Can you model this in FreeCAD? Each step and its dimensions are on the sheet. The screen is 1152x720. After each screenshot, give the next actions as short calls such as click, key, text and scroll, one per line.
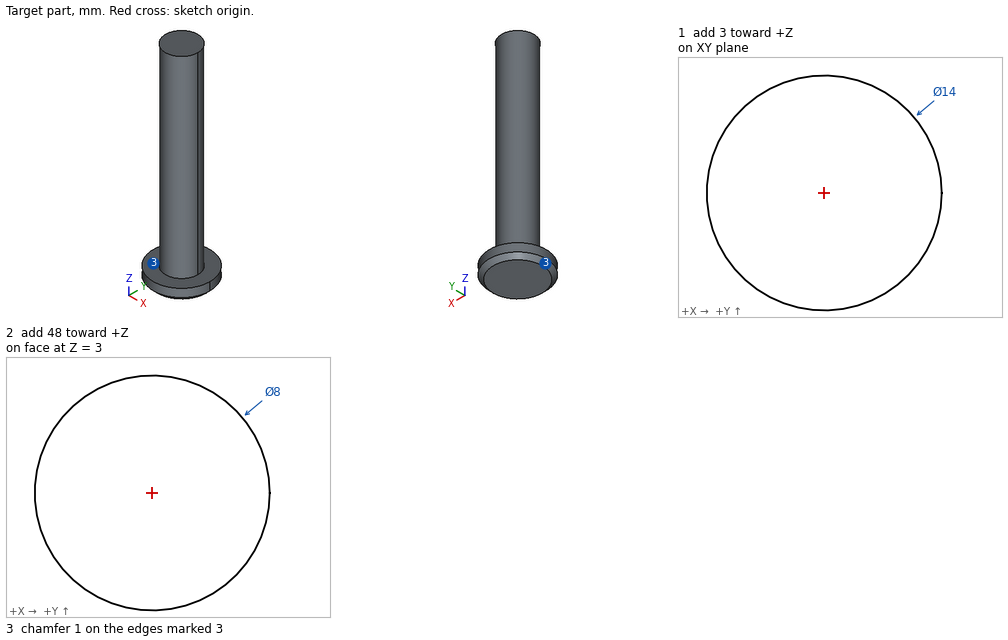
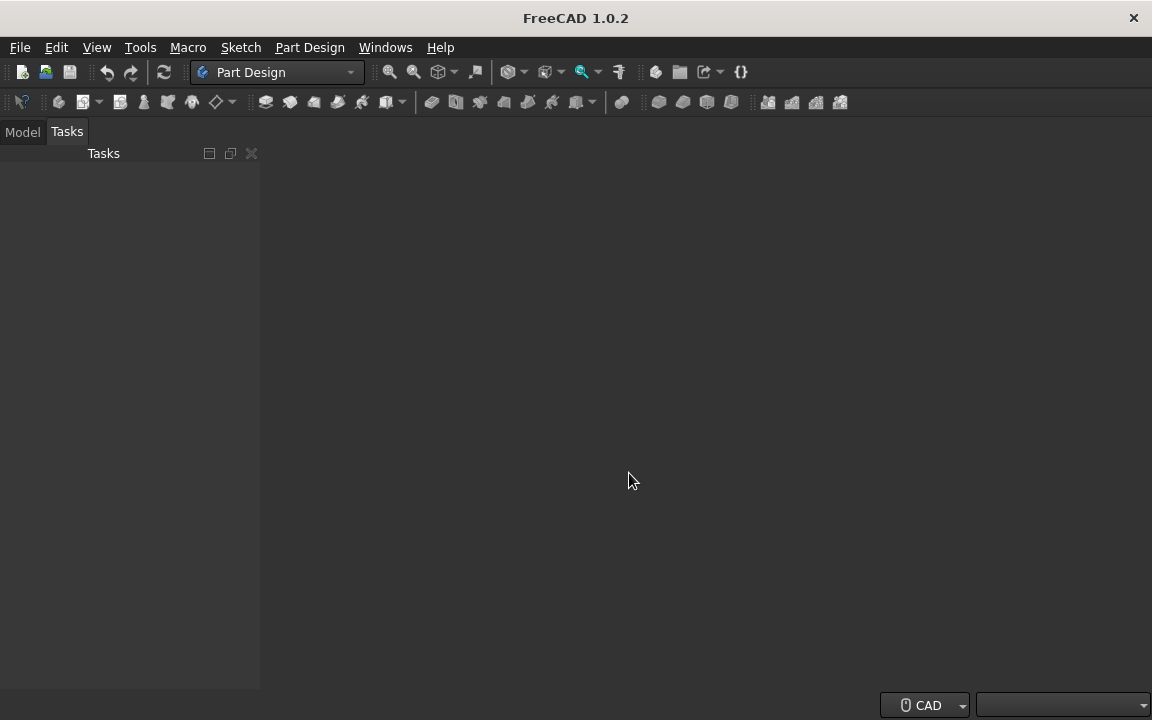
click(22, 72)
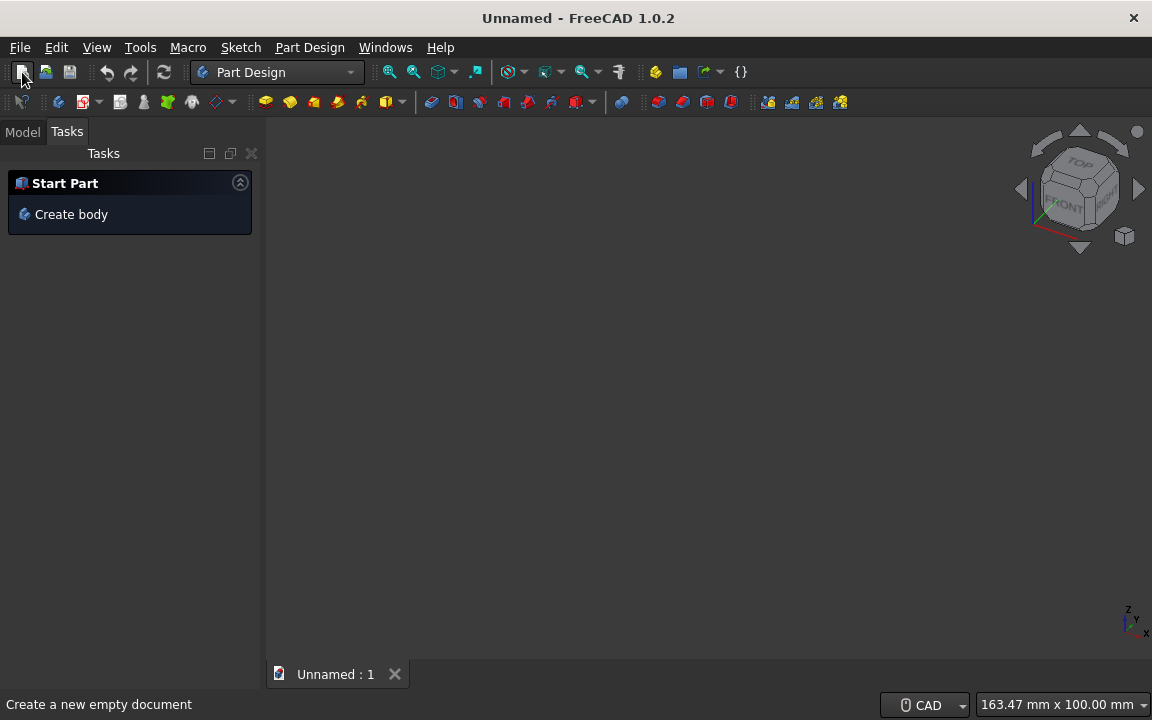
click(84, 102)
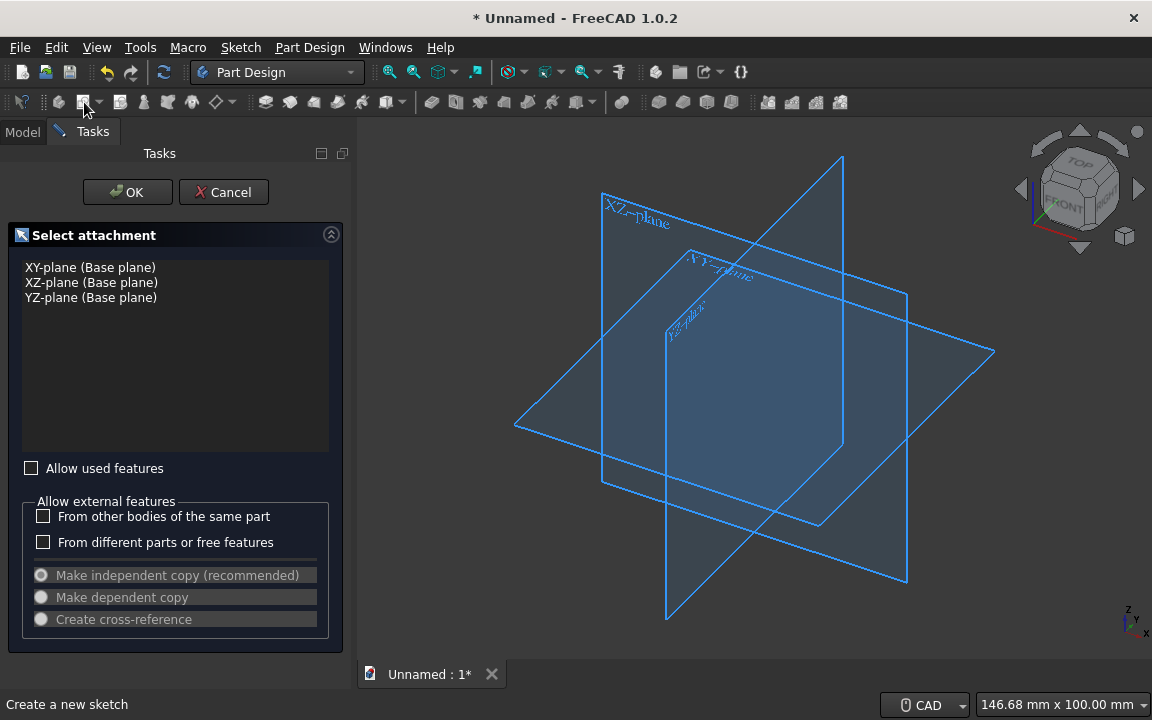
click(82, 268)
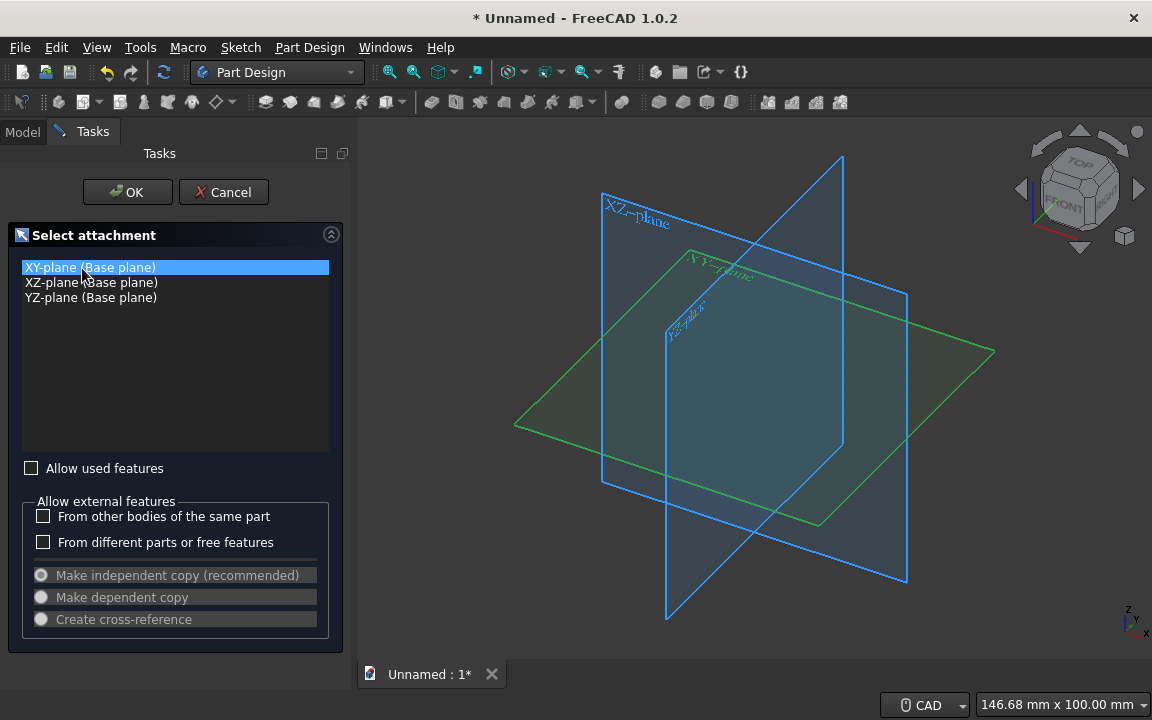
click(128, 192)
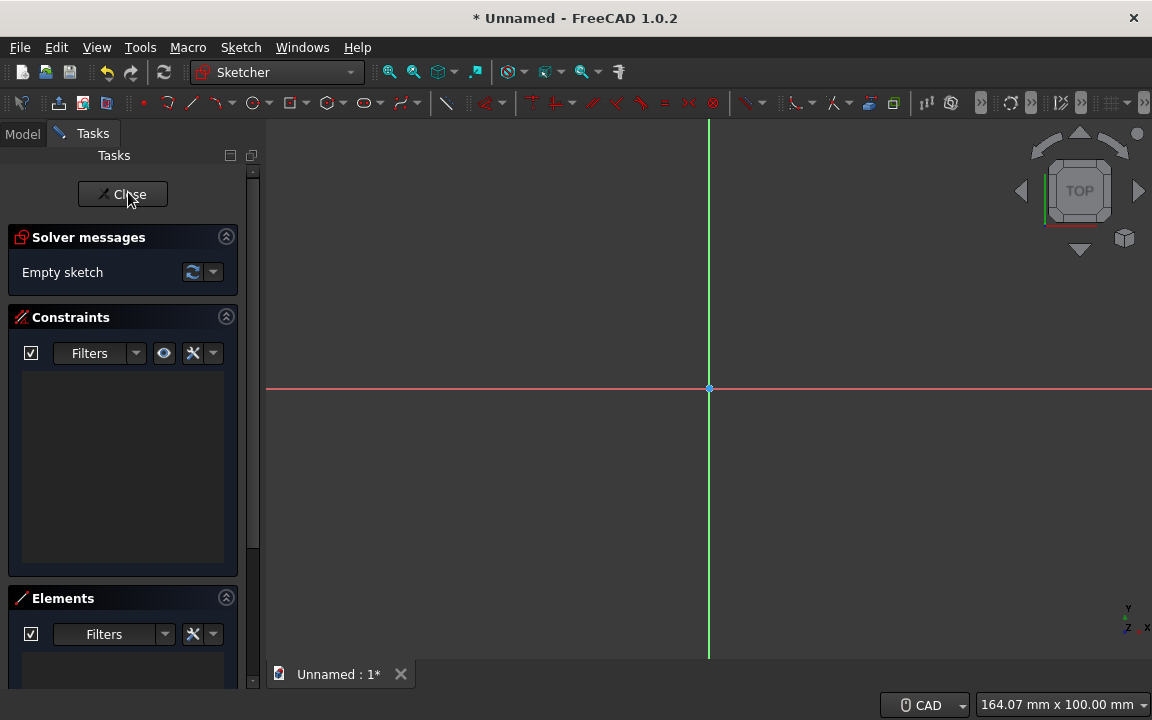
scroll(726, 389, up, 8)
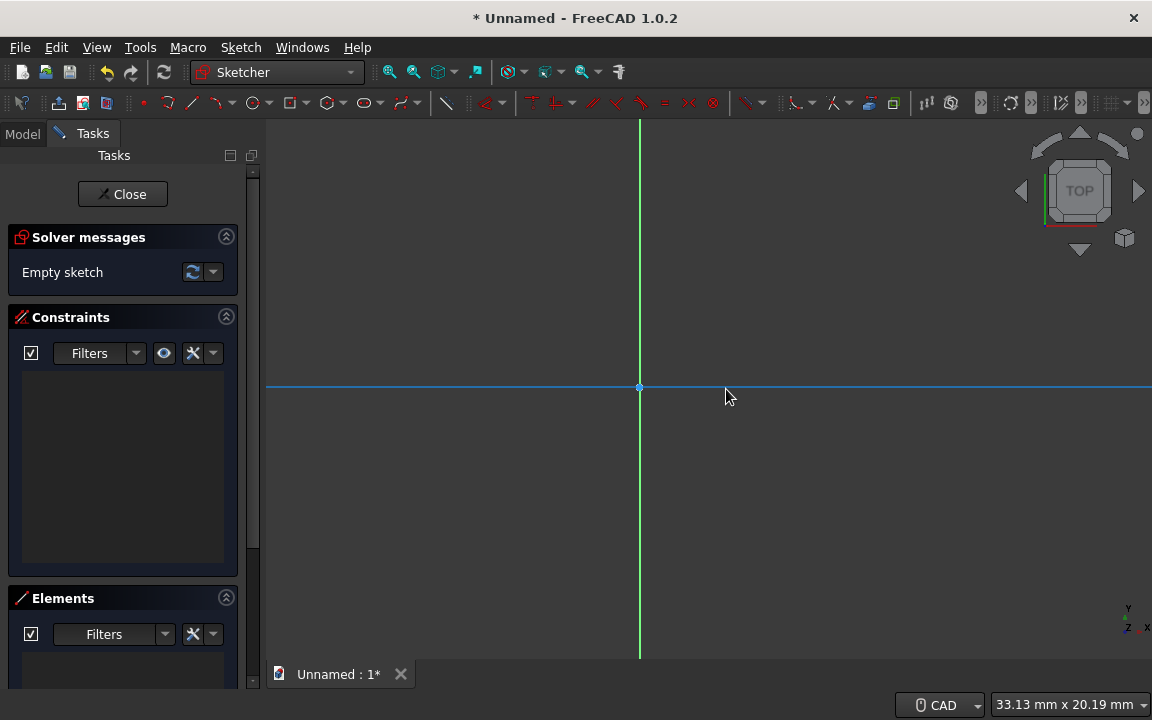
click(254, 104)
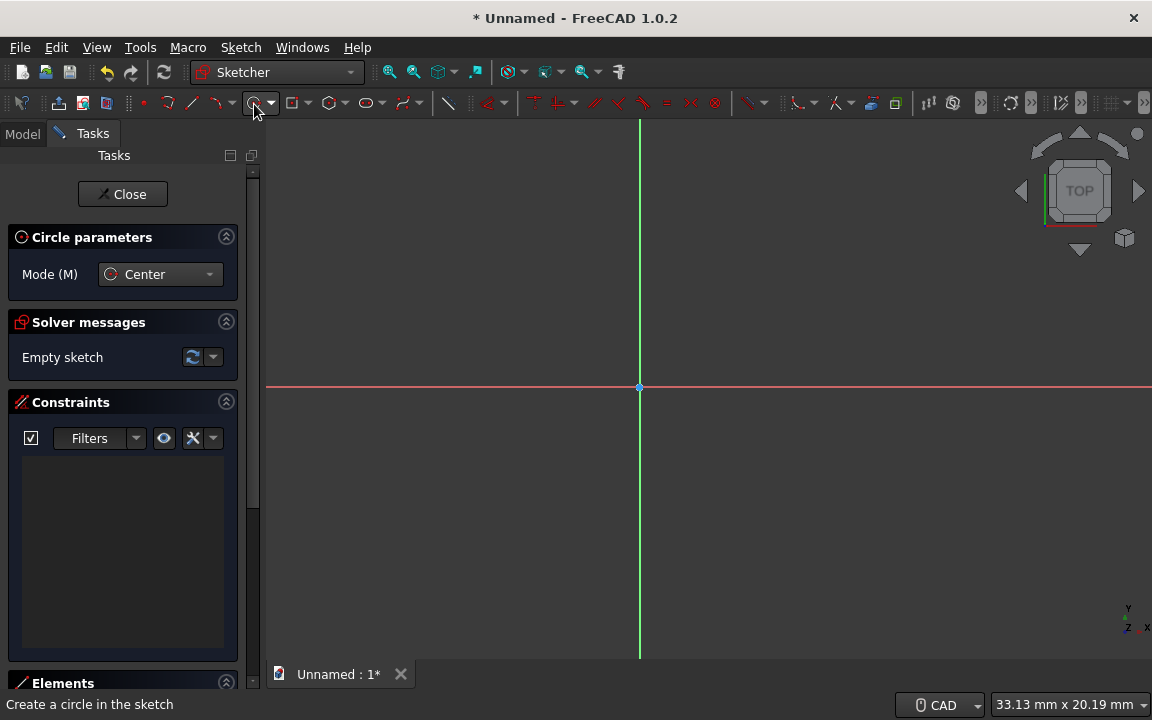
click(640, 387)
click(772, 255)
key(Escape)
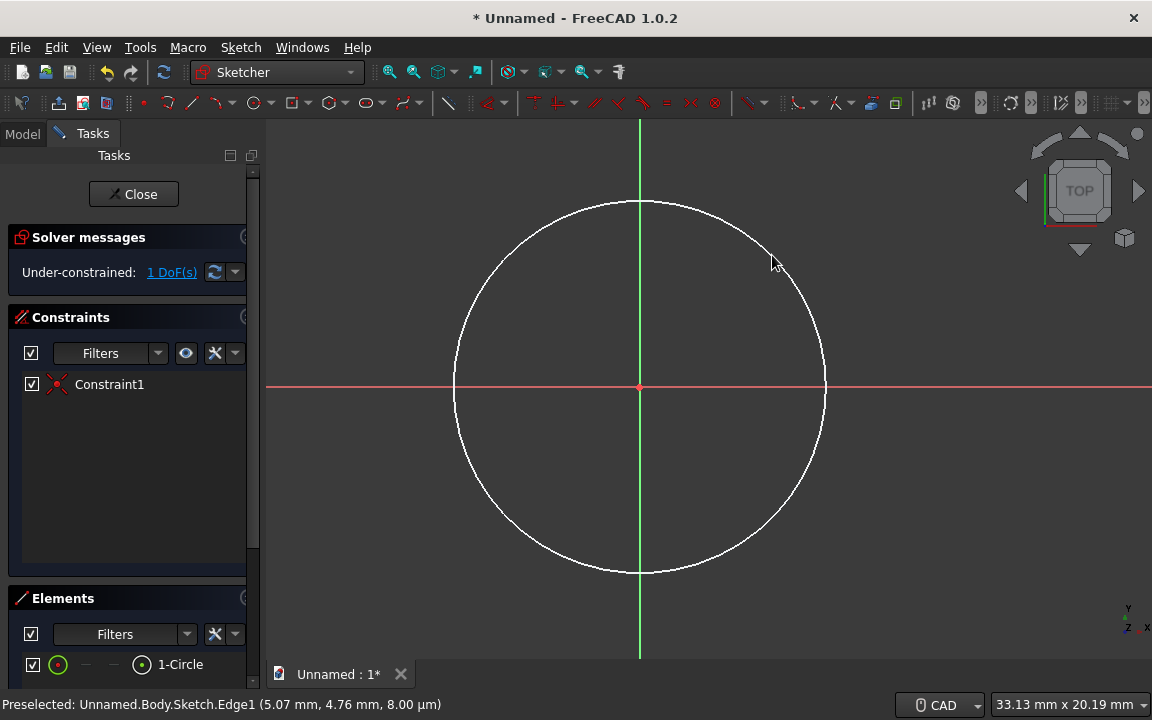
click(771, 255)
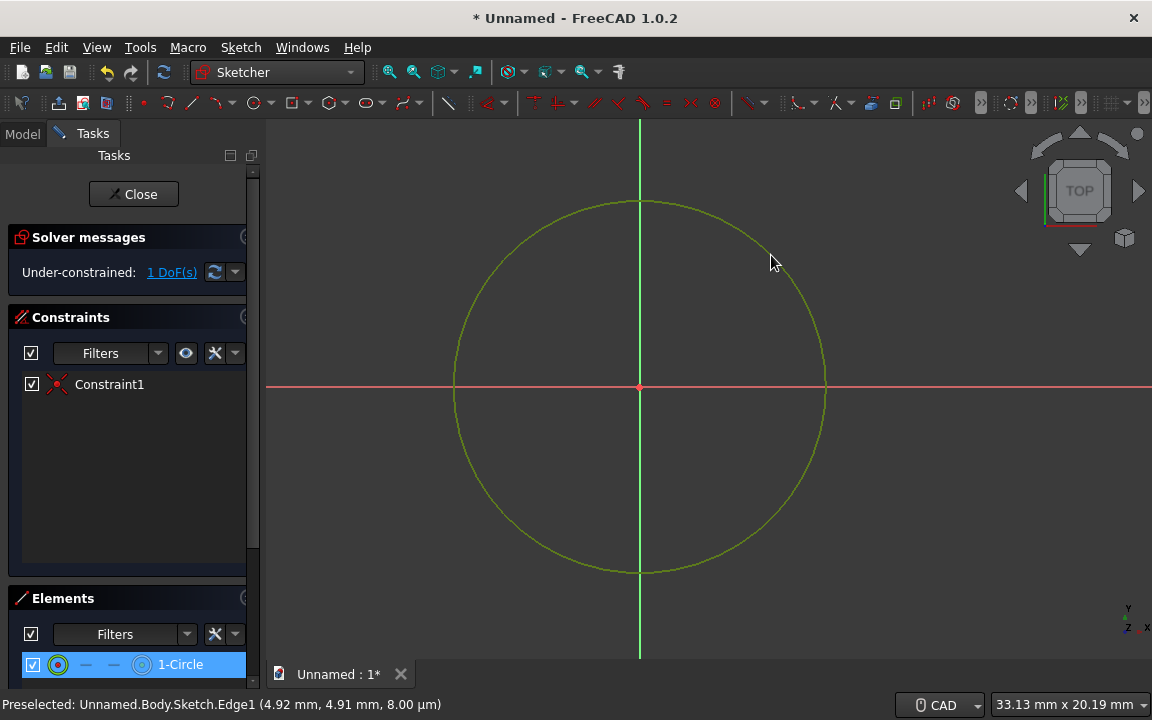
key(k)
key(o)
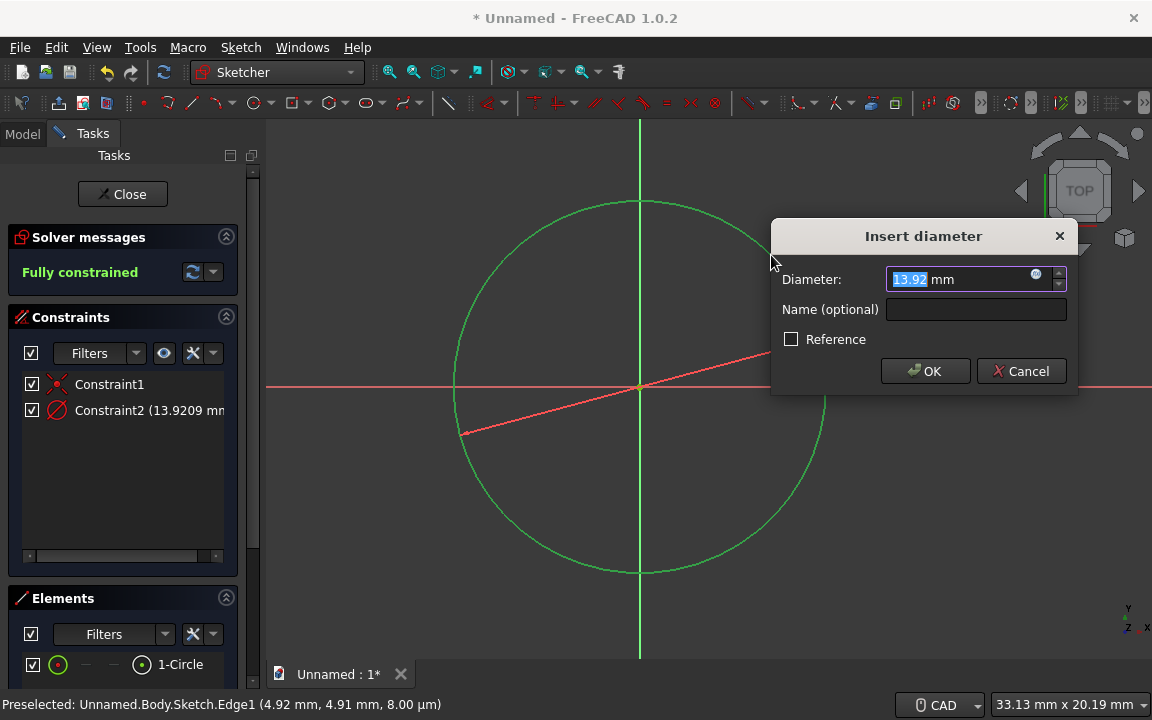
text(14)
key(Return)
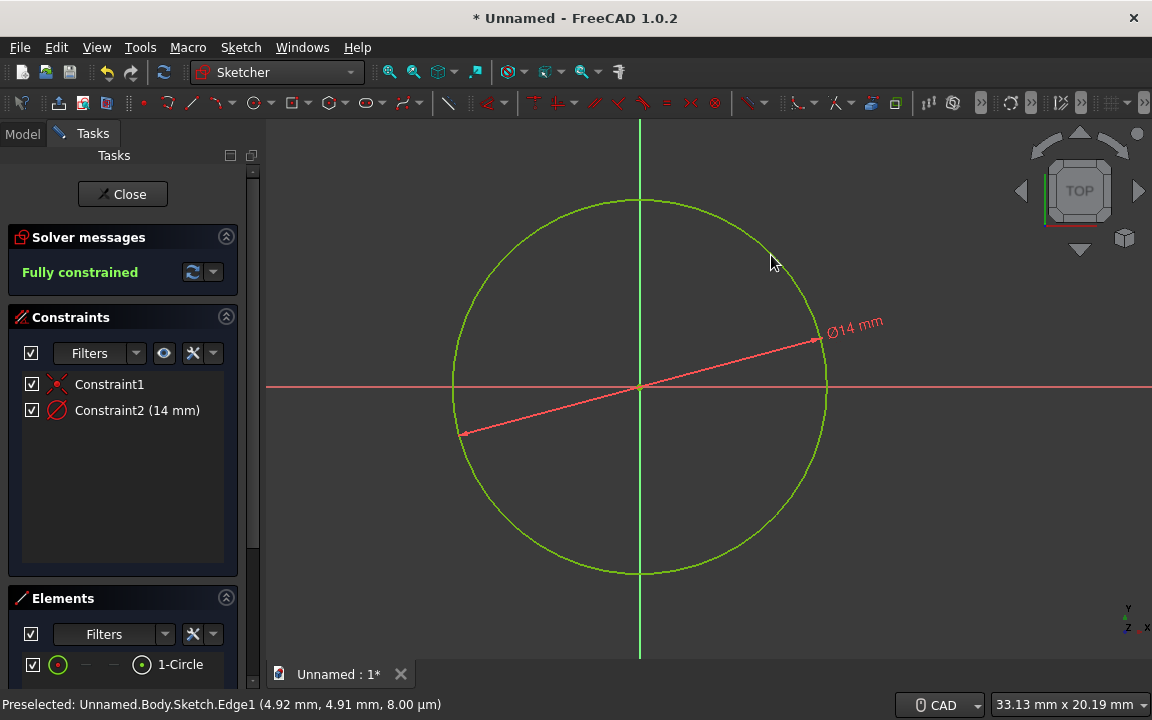
click(123, 194)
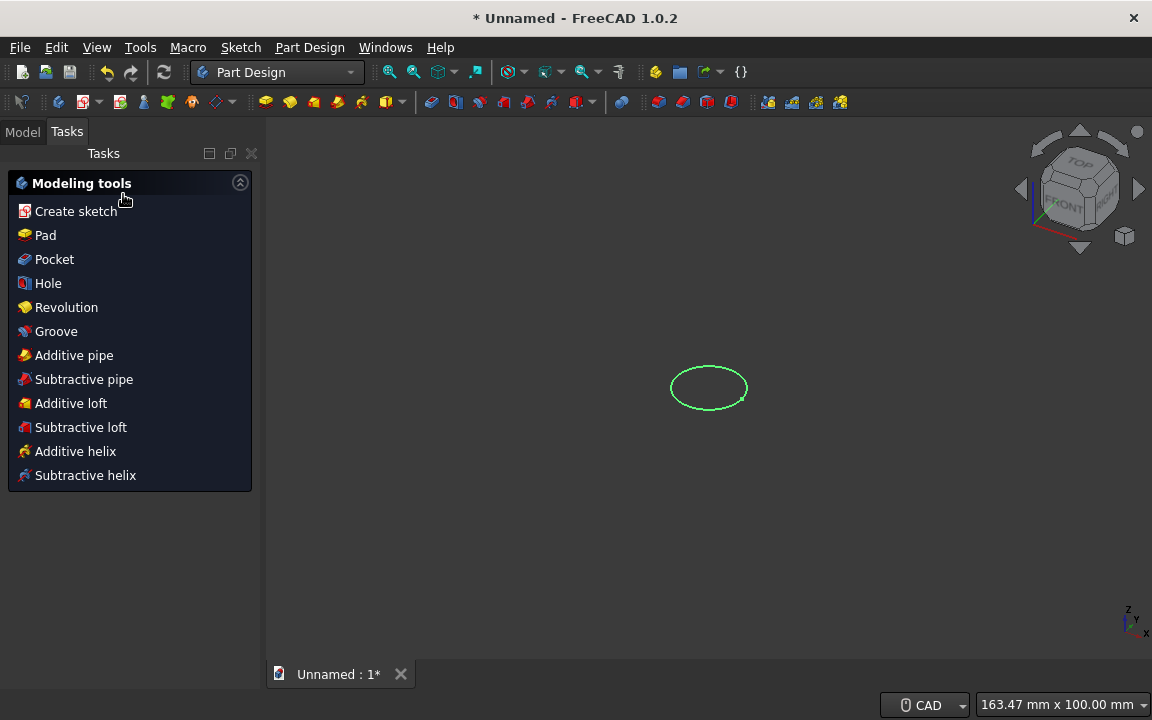
click(266, 102)